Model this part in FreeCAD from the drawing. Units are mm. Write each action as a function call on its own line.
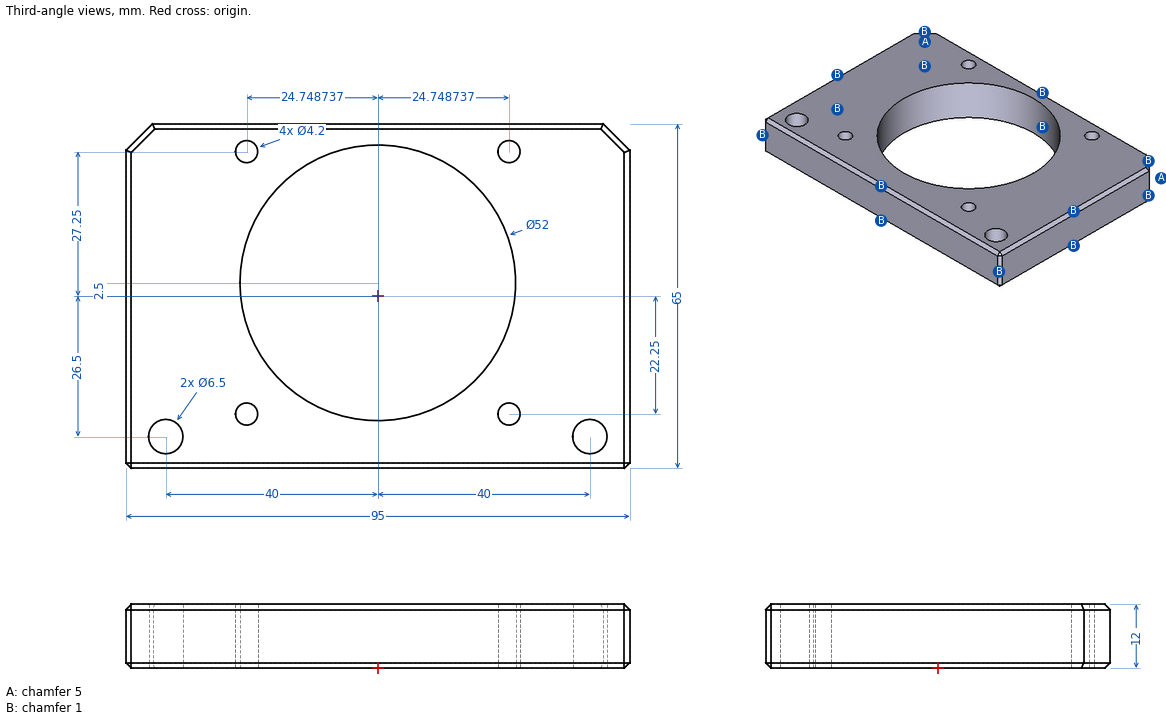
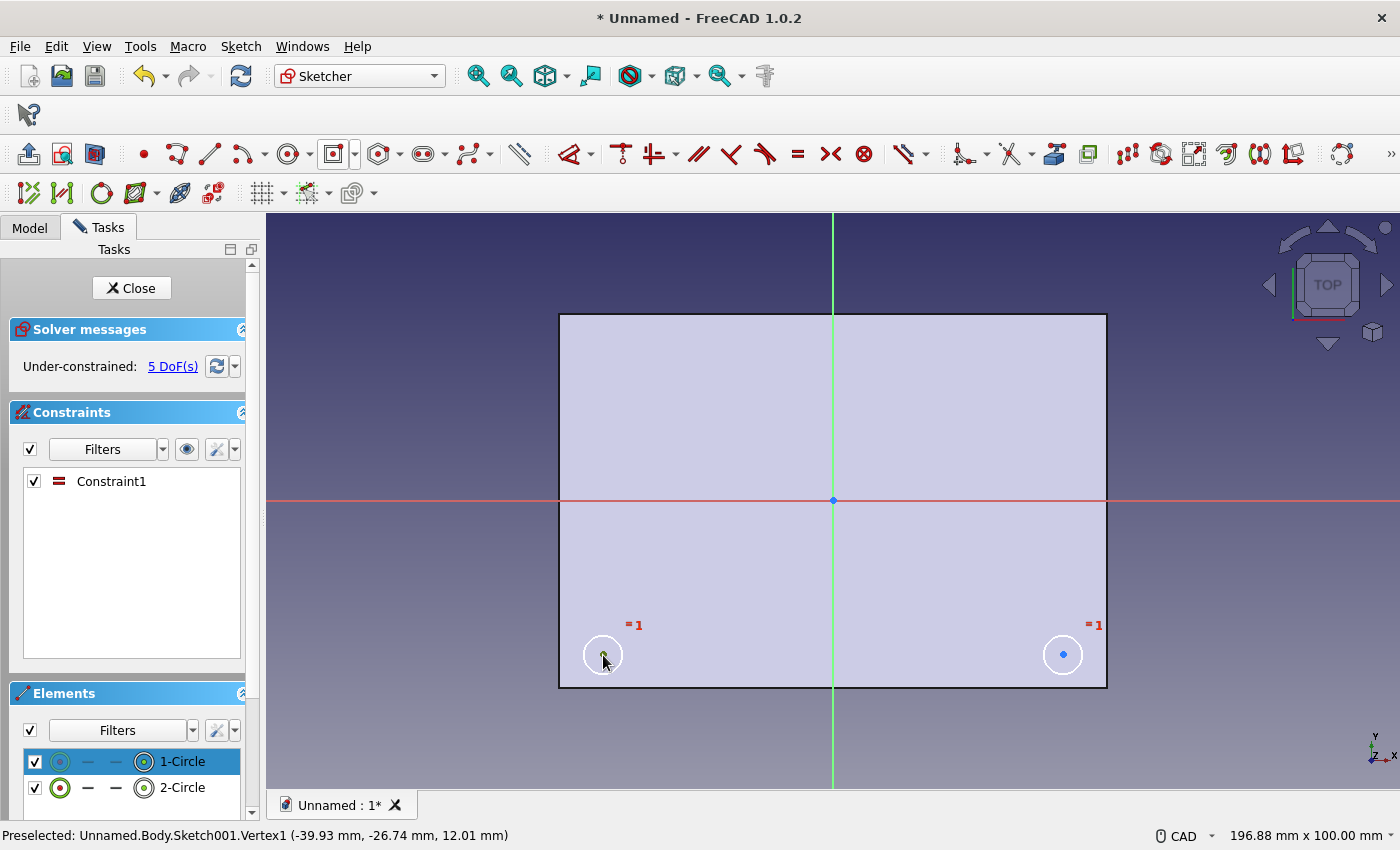
click(1063, 655)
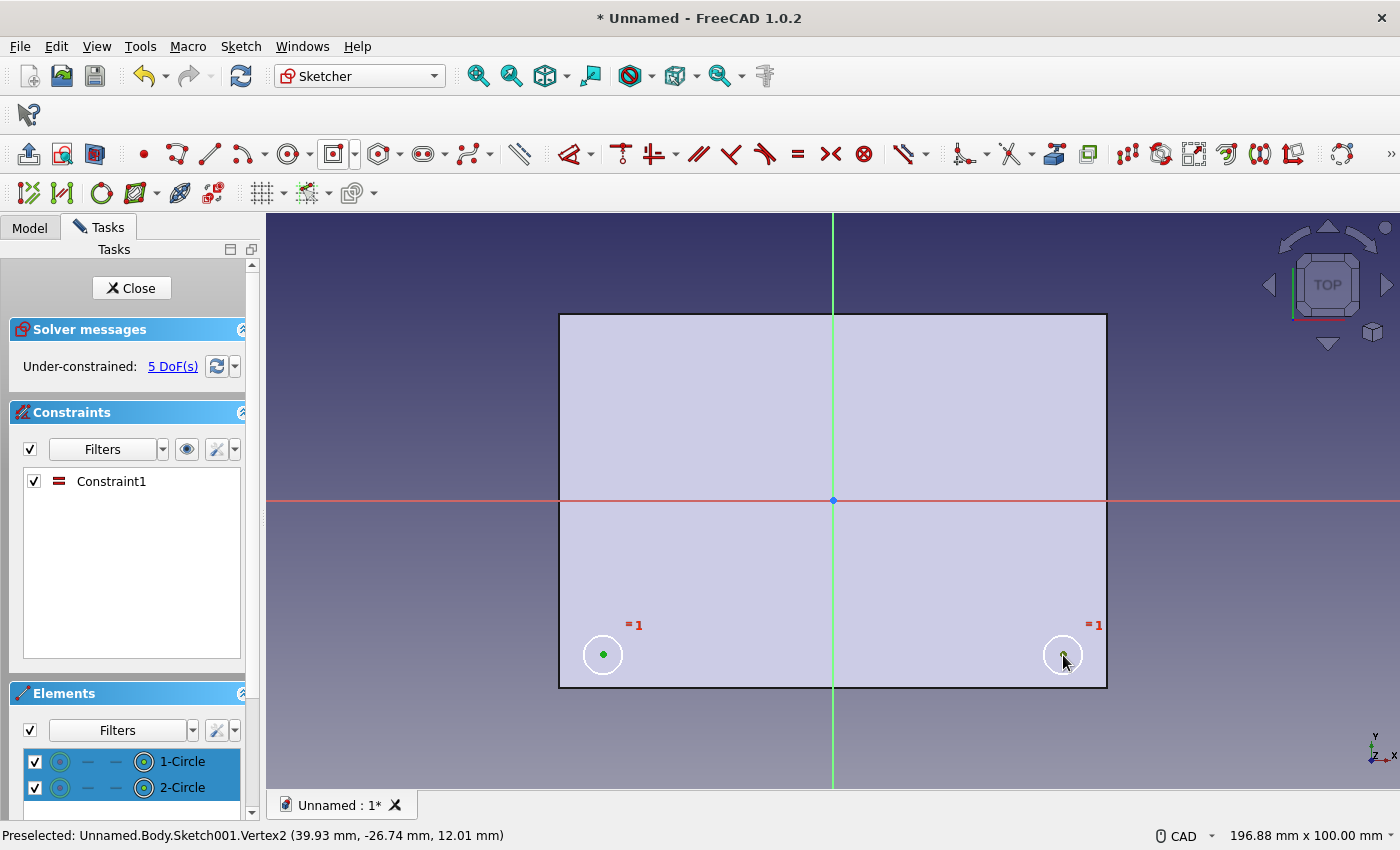
click(676, 154)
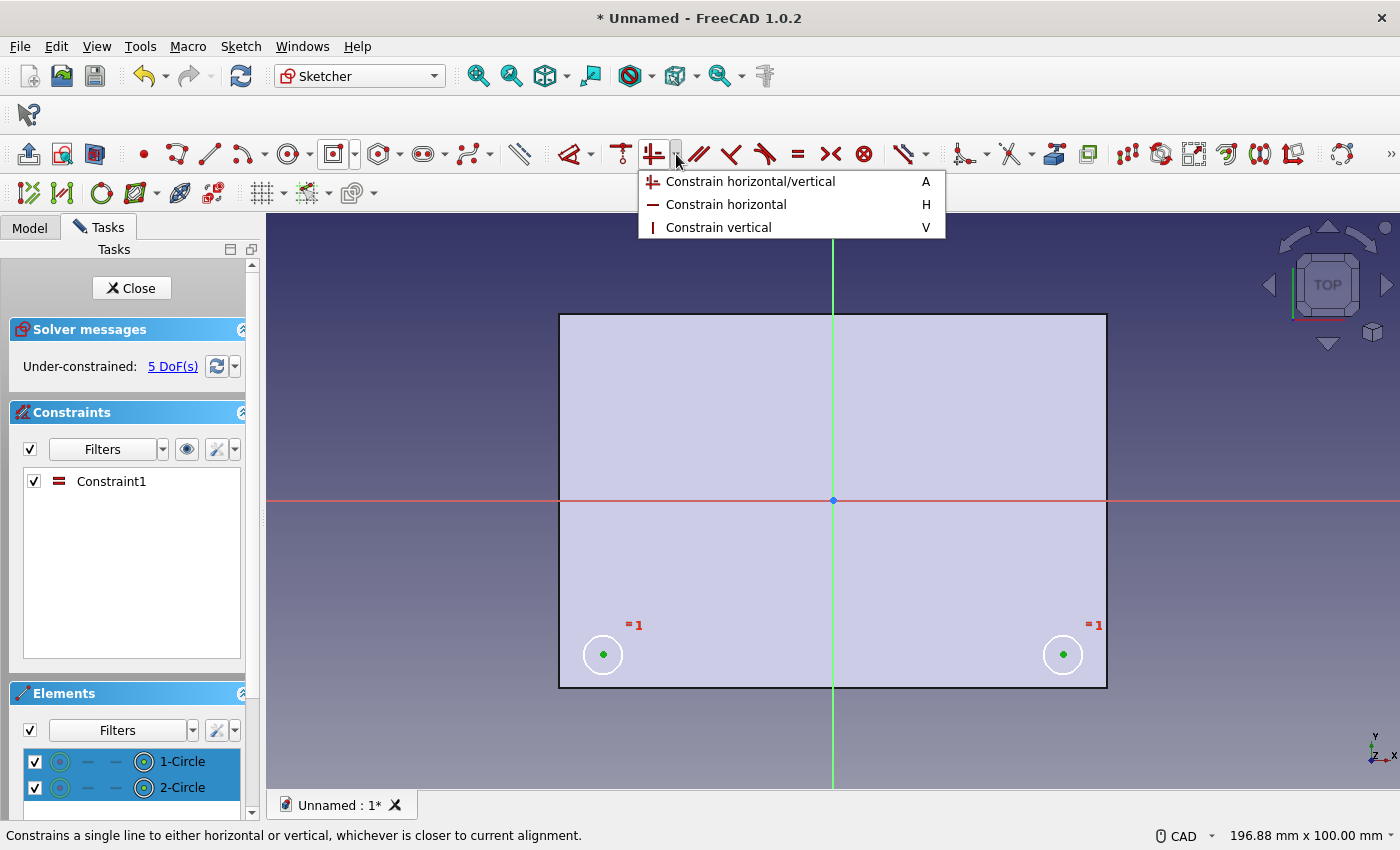
click(792, 204)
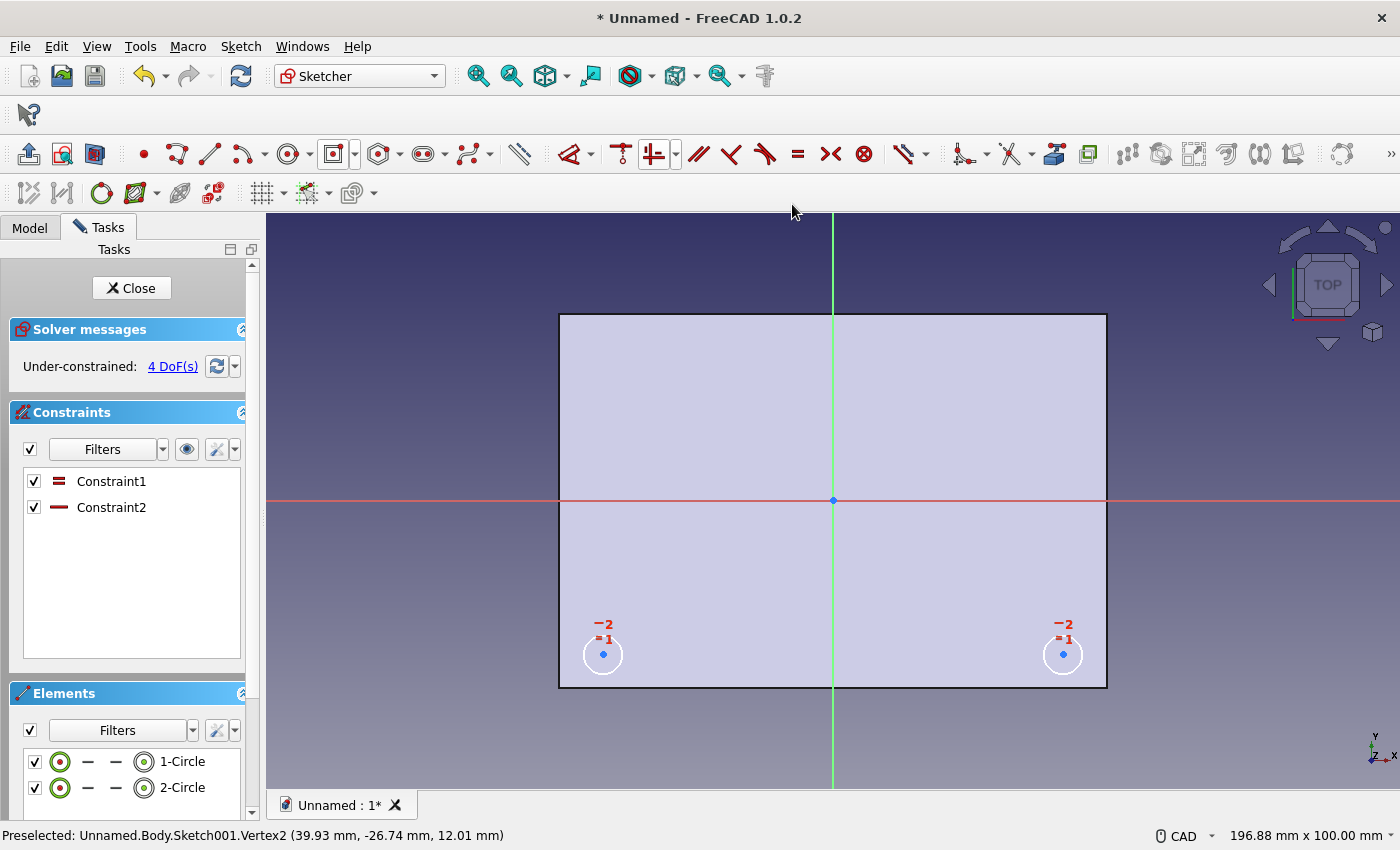
key(d)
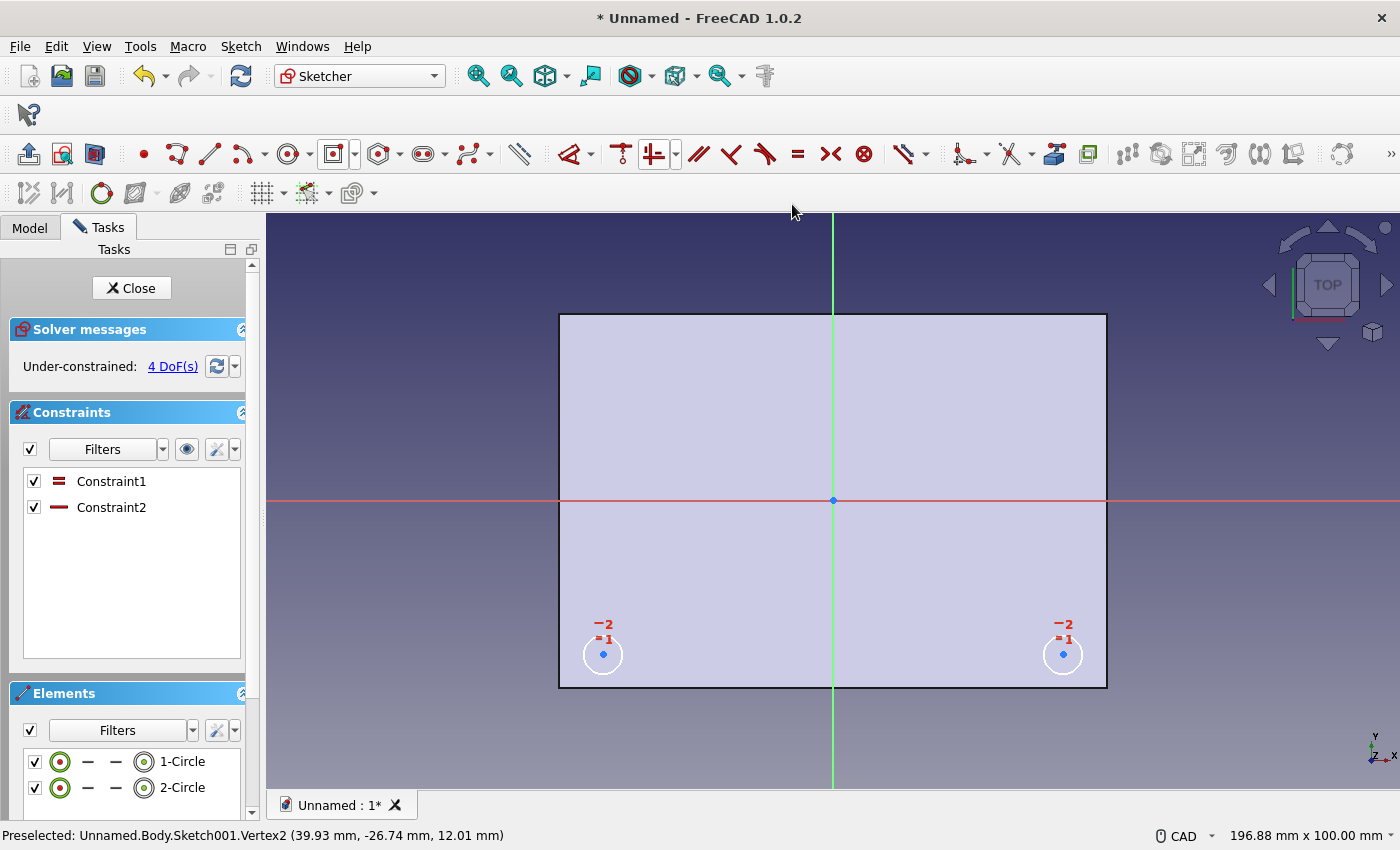
click(616, 641)
click(638, 618)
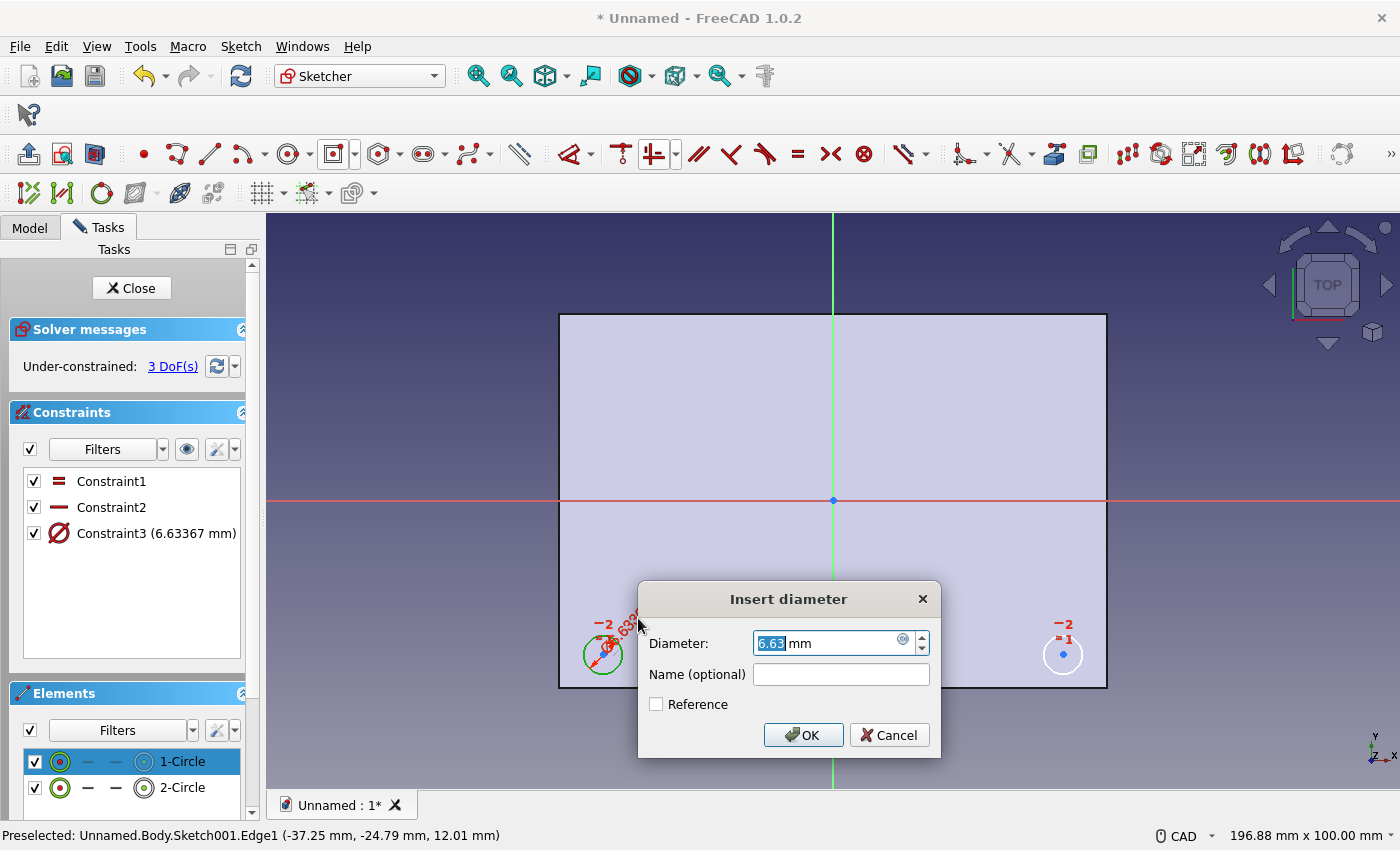
text(6.5)
key(Return)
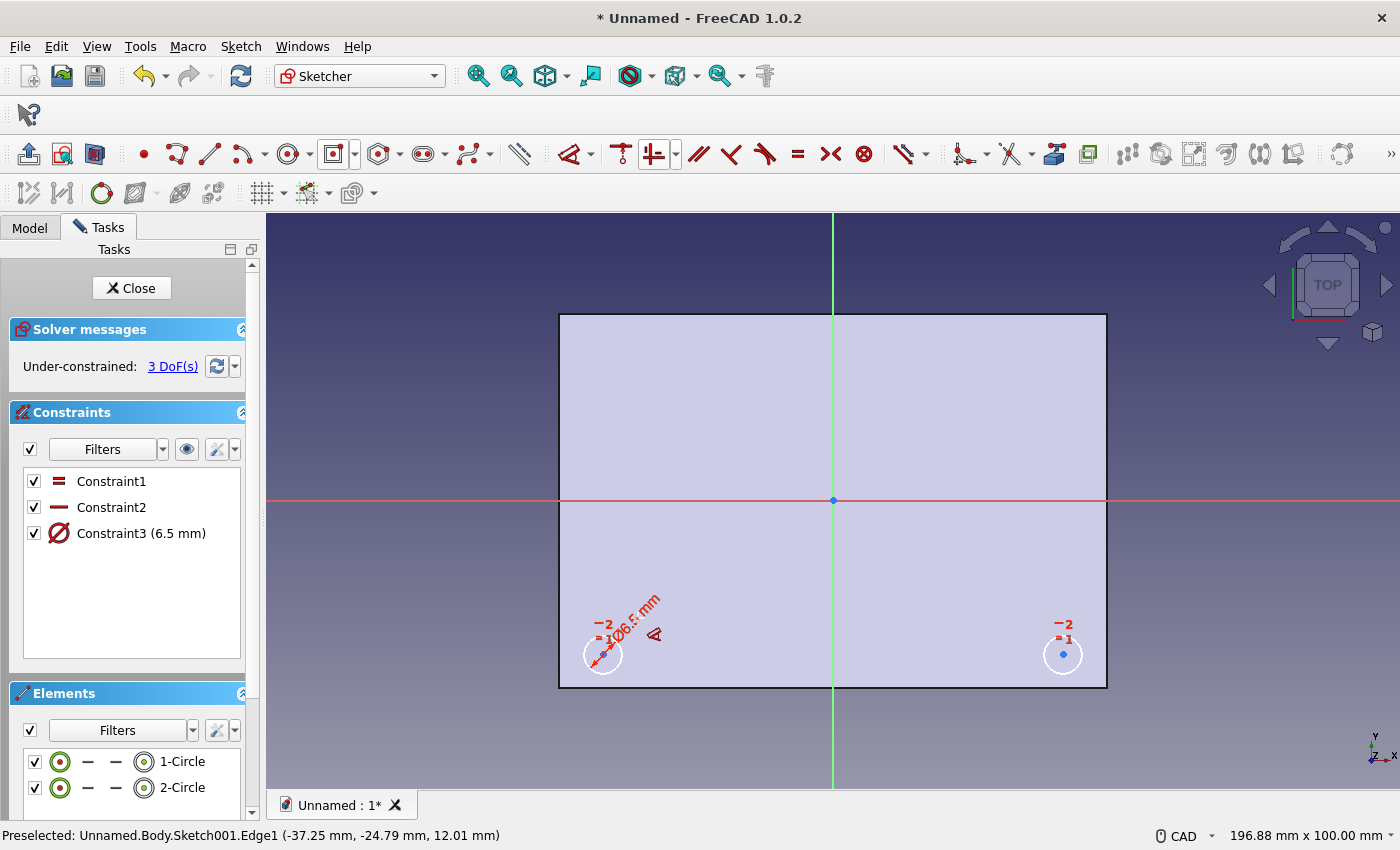
click(603, 655)
click(718, 467)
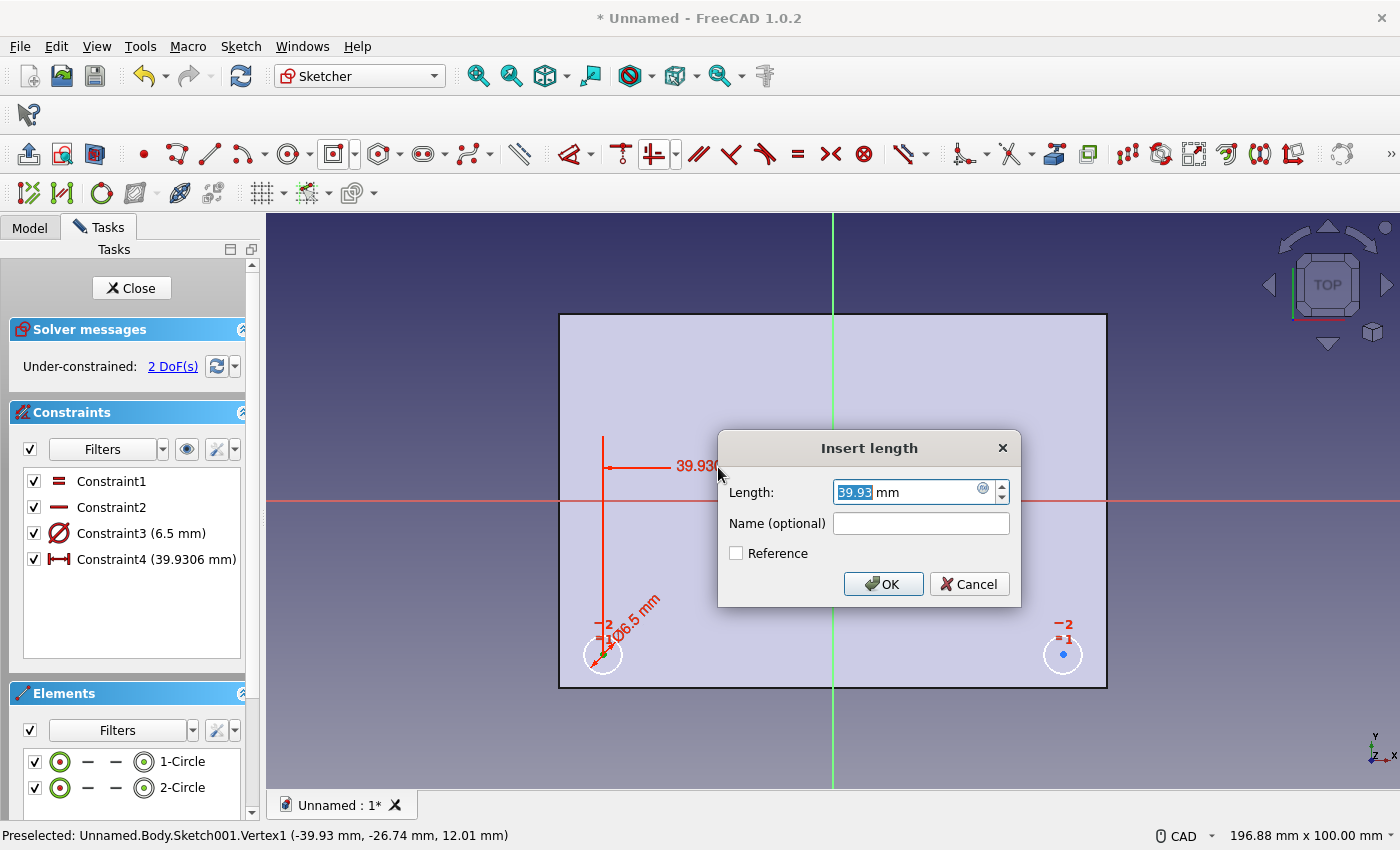
text(40)
key(Return)